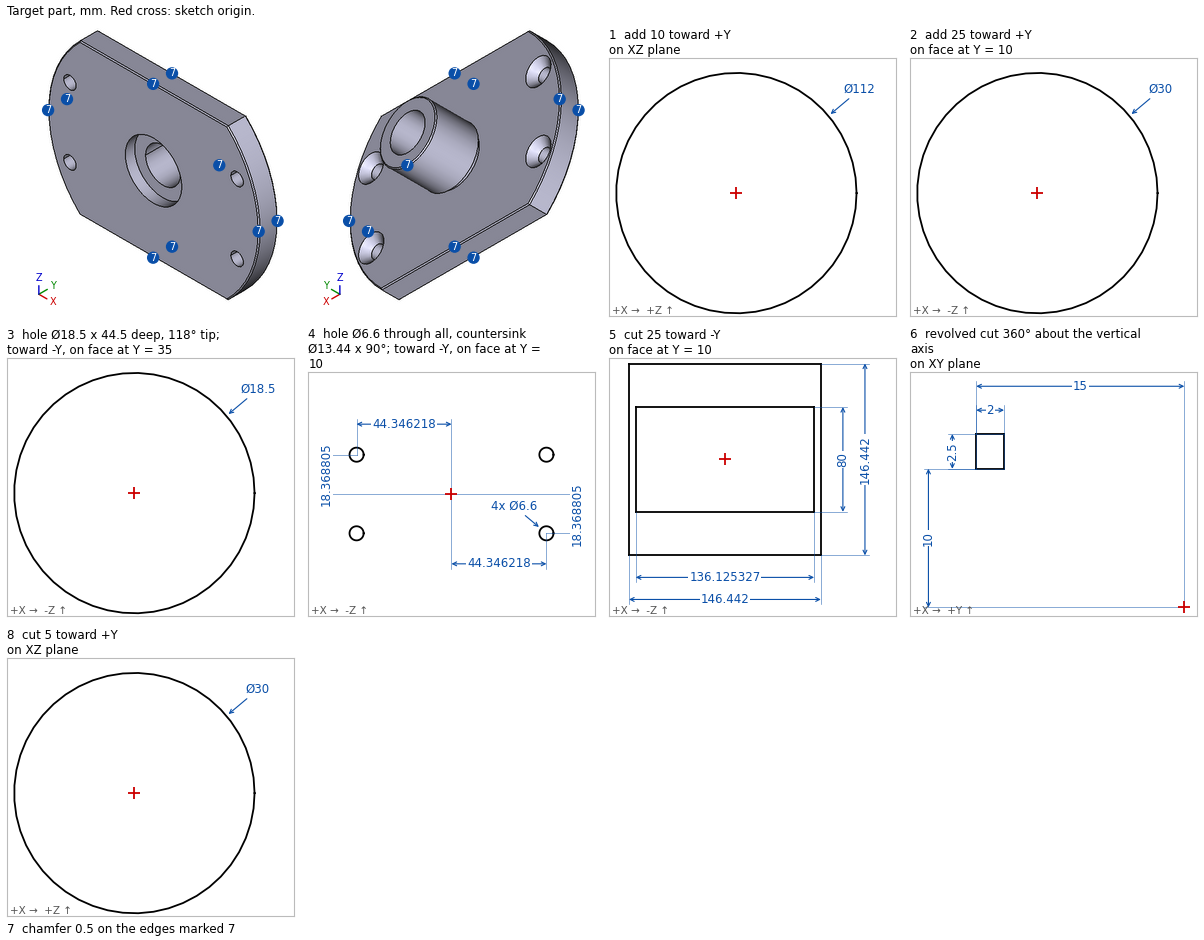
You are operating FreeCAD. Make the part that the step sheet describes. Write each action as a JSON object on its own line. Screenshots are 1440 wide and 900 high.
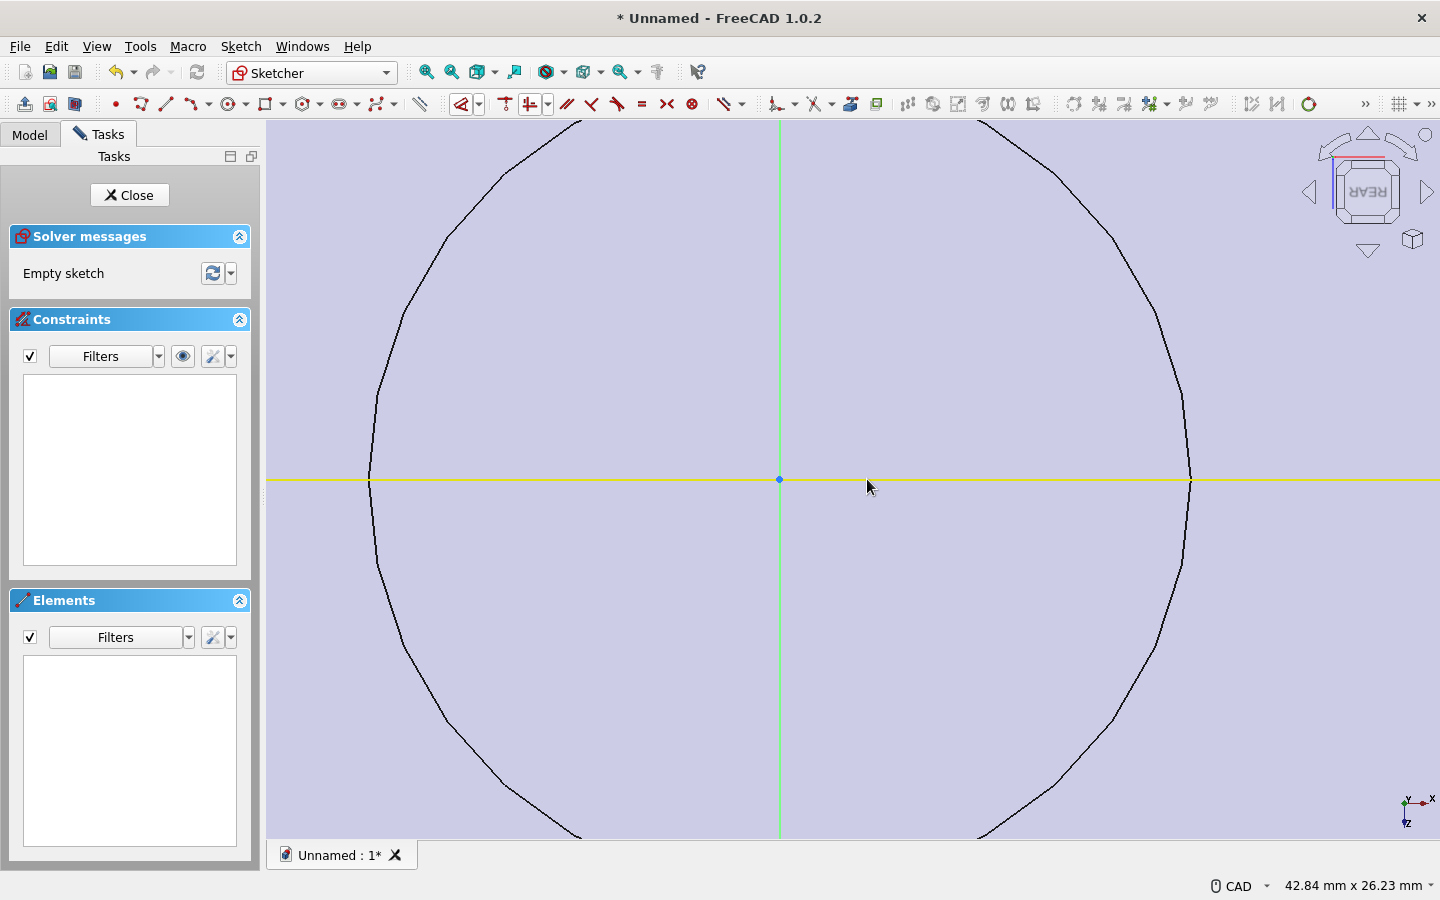
{"action": "key", "text": "g c"}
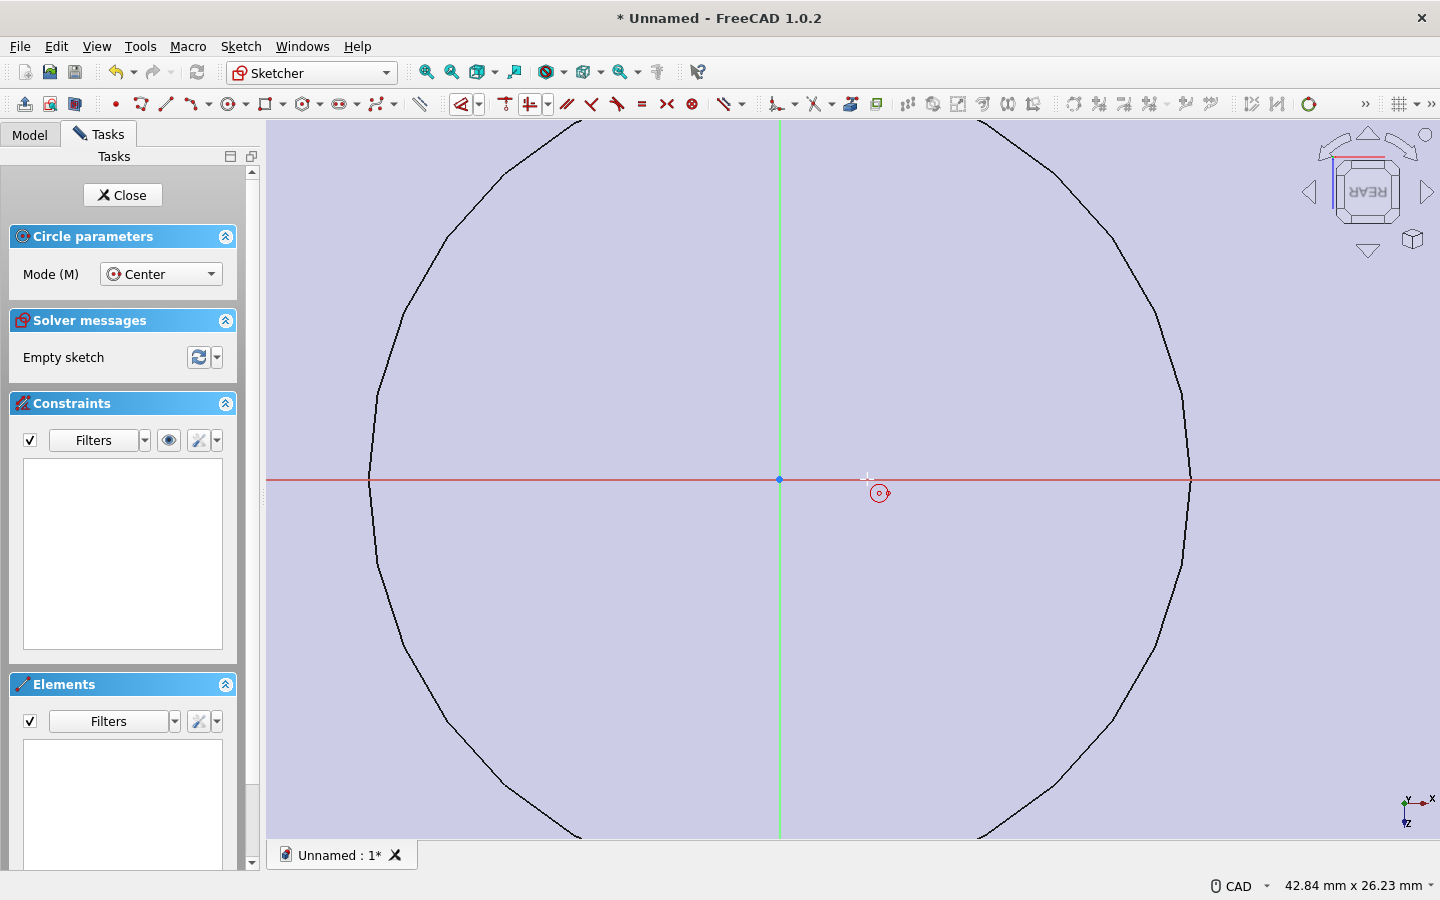
{"action": "left_click", "coordinate": [780, 479]}
{"action": "mouse_move", "coordinate": [959, 300]}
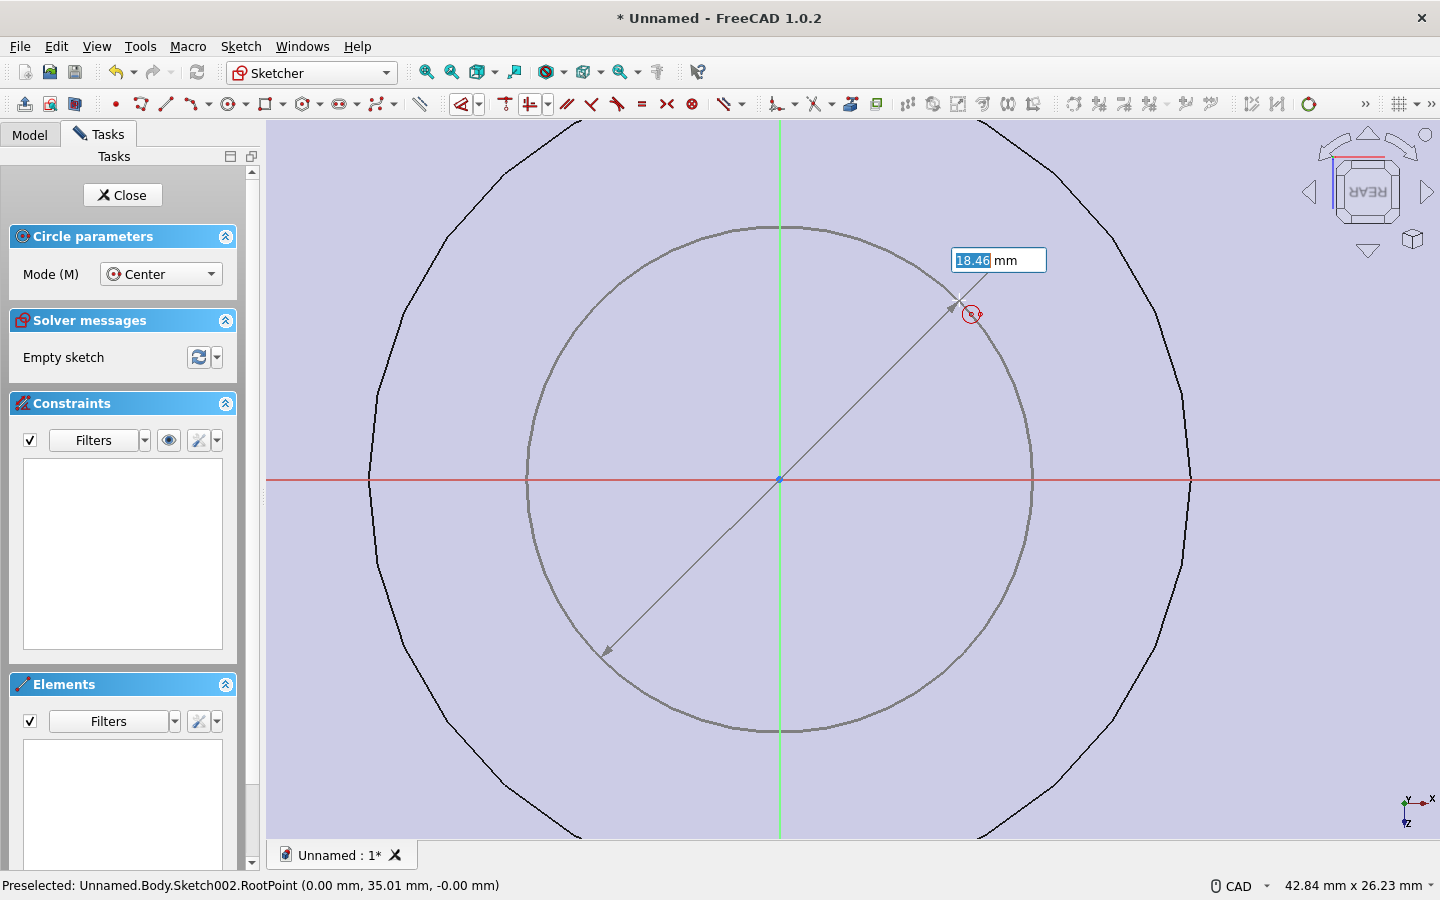
{"action": "type", "text": "18.5"}
{"action": "key", "text": "Return"}
{"action": "key", "text": "Escape"}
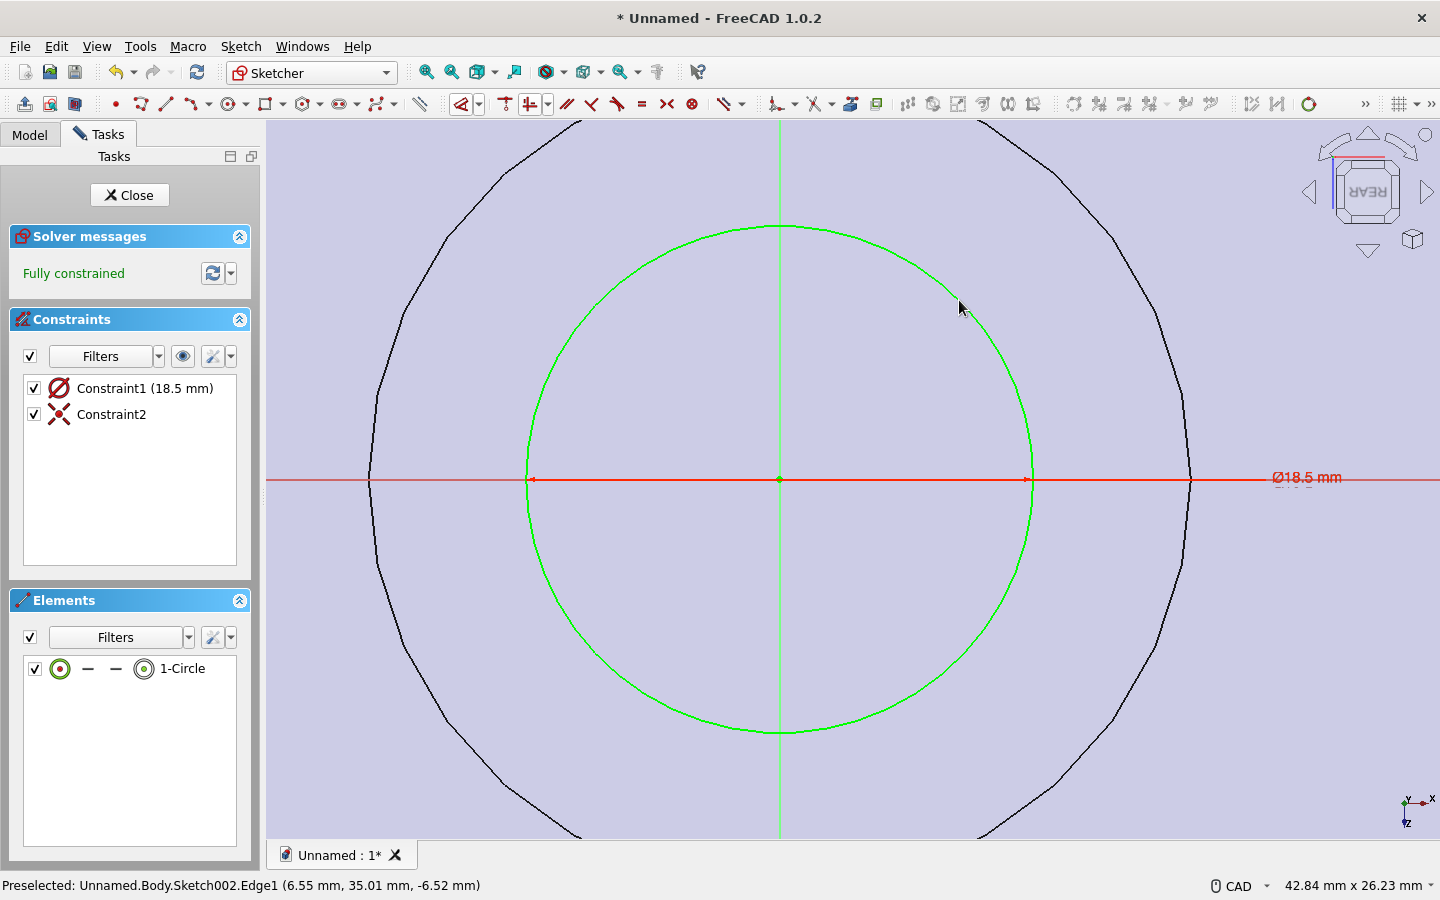
{"action": "left_click", "coordinate": [130, 195]}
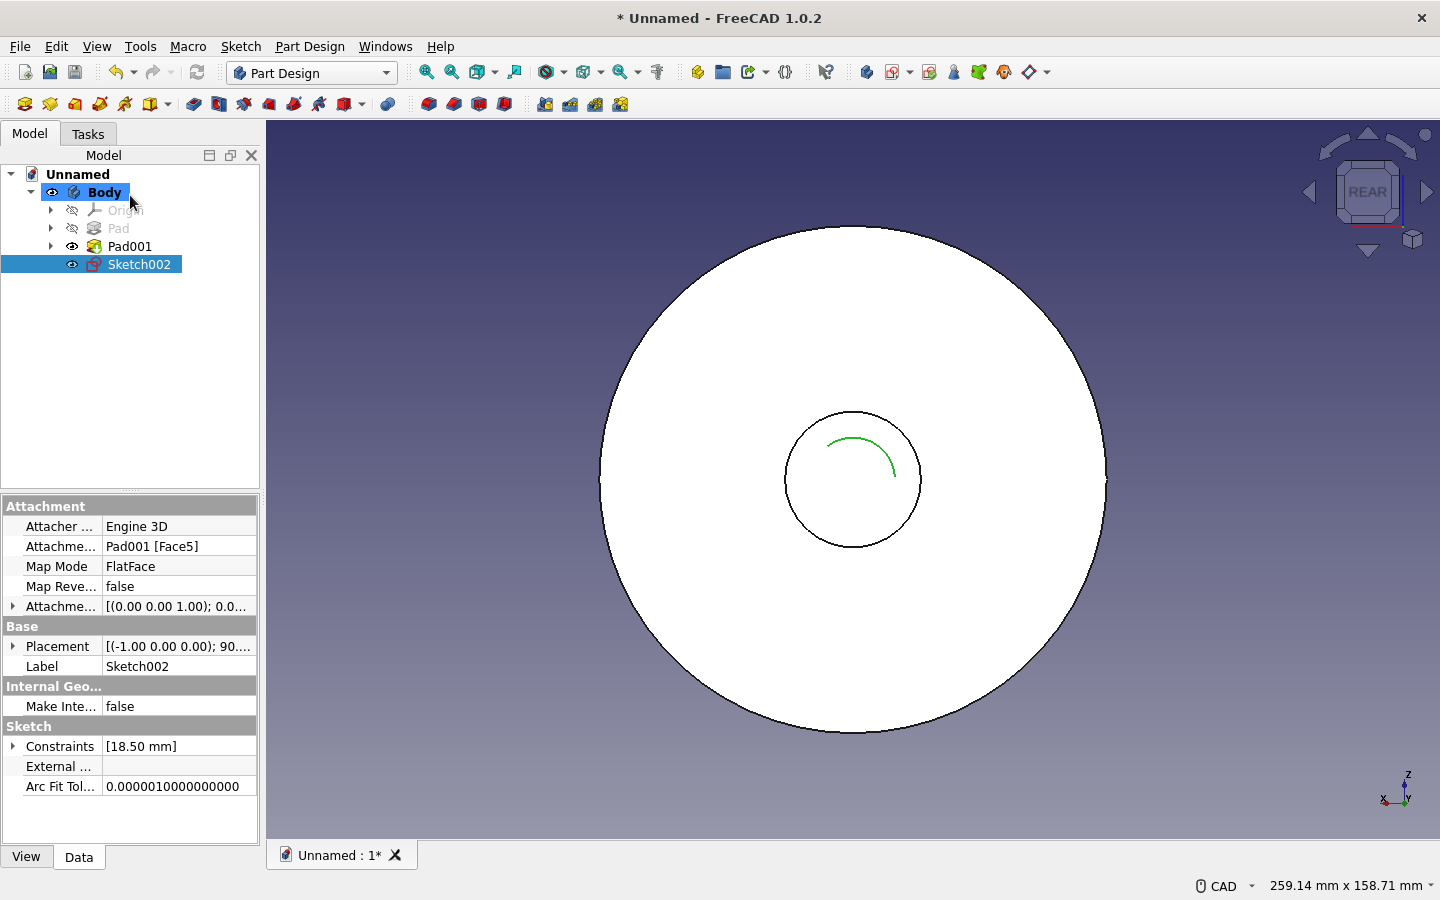
{"action": "left_click", "coordinate": [219, 104]}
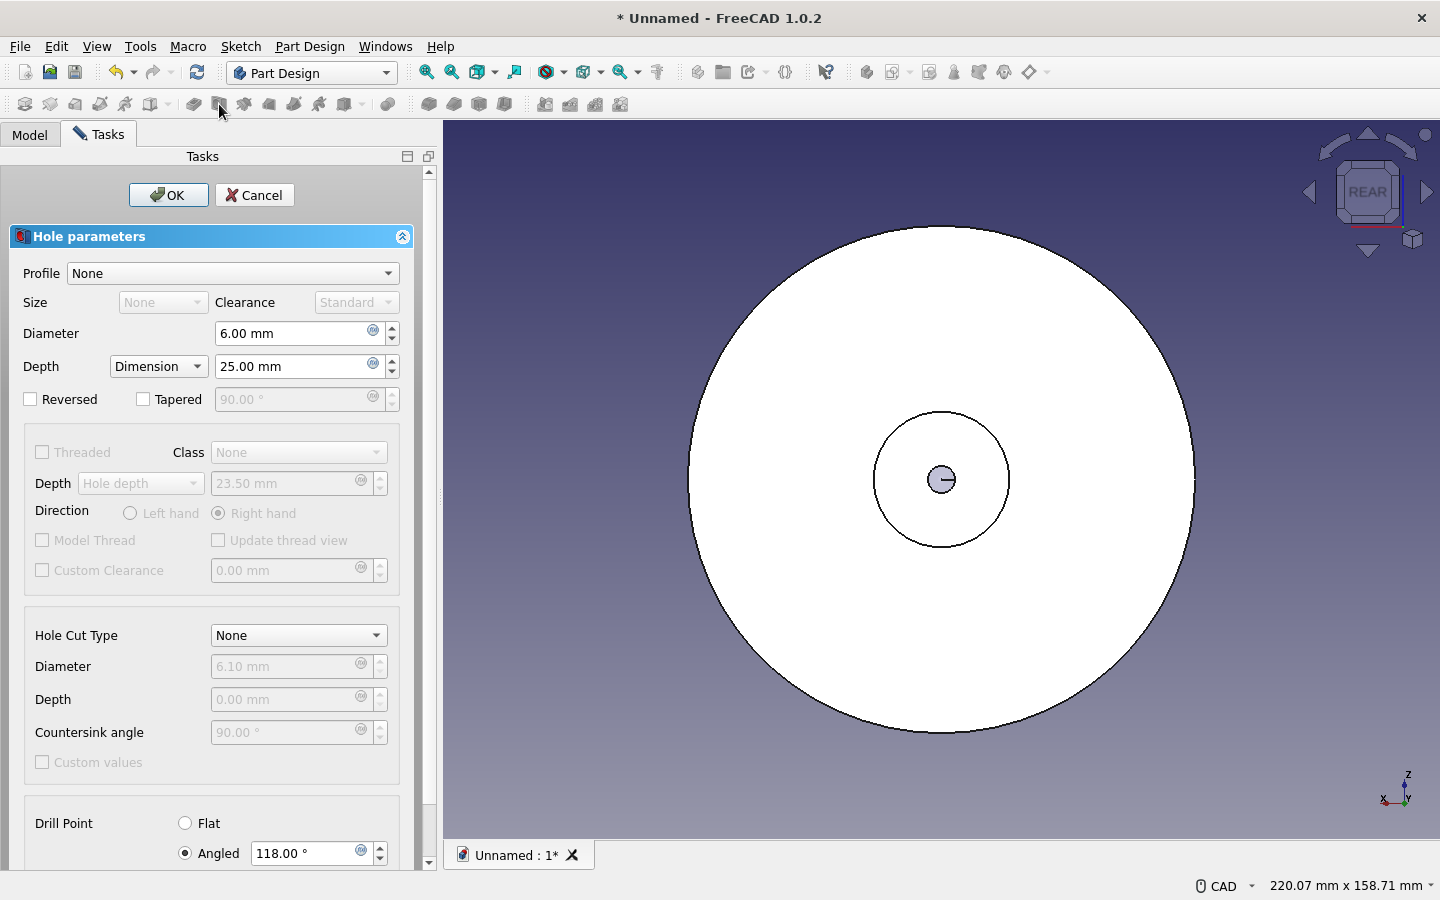
{"action": "triple_click", "coordinate": [300, 334]}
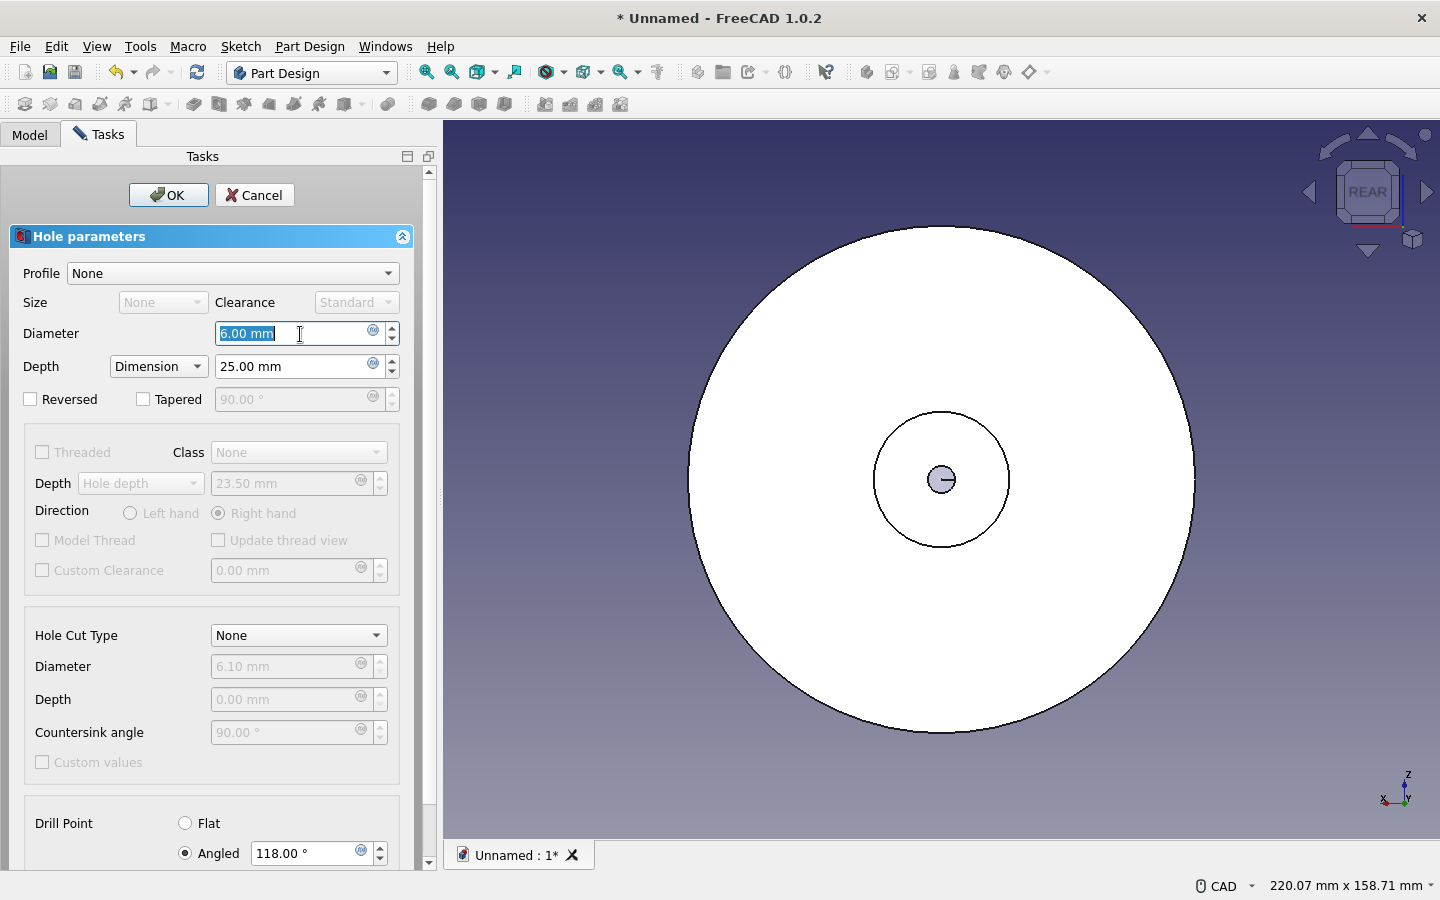
{"action": "type", "text": "18.5"}
{"action": "key", "text": "Tab"}